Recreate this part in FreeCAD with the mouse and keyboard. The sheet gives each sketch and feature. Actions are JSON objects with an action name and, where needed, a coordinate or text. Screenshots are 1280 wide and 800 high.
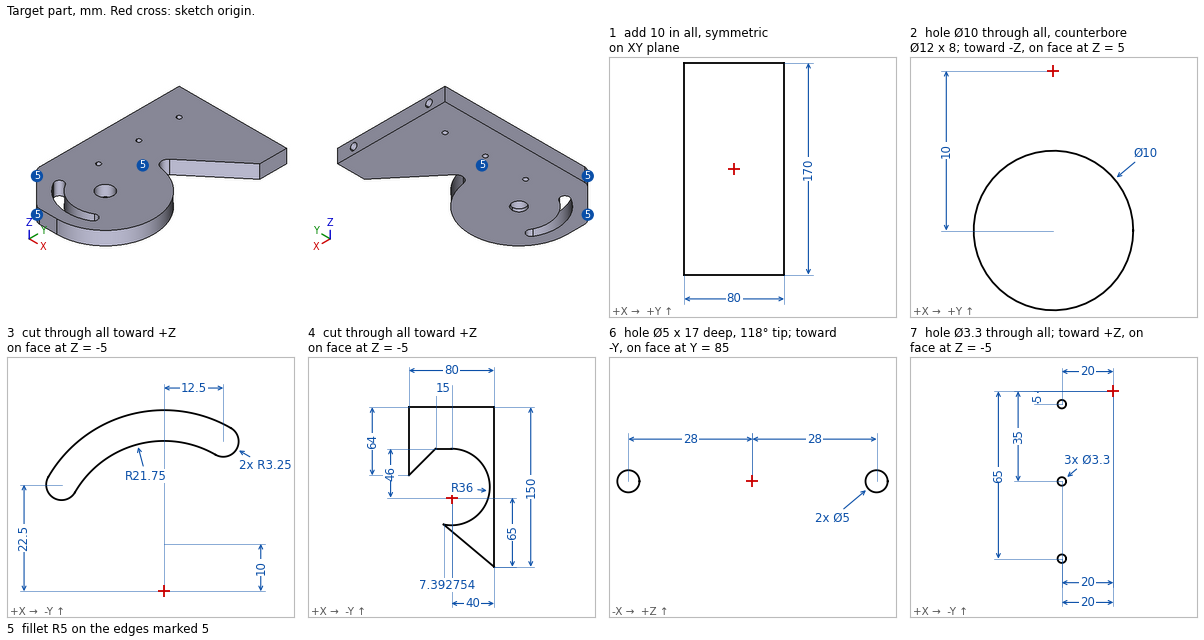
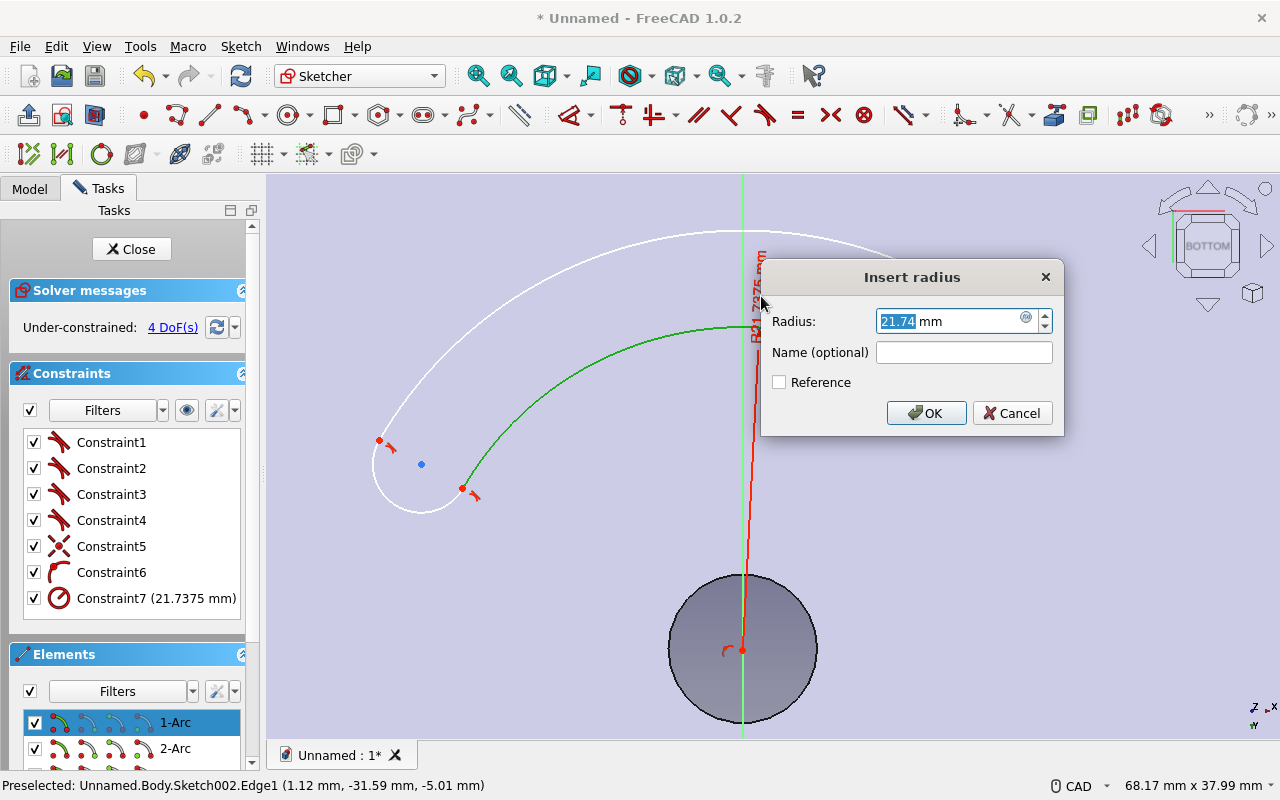
{"action": "type", "text": "21.75"}
{"action": "key", "text": "Return"}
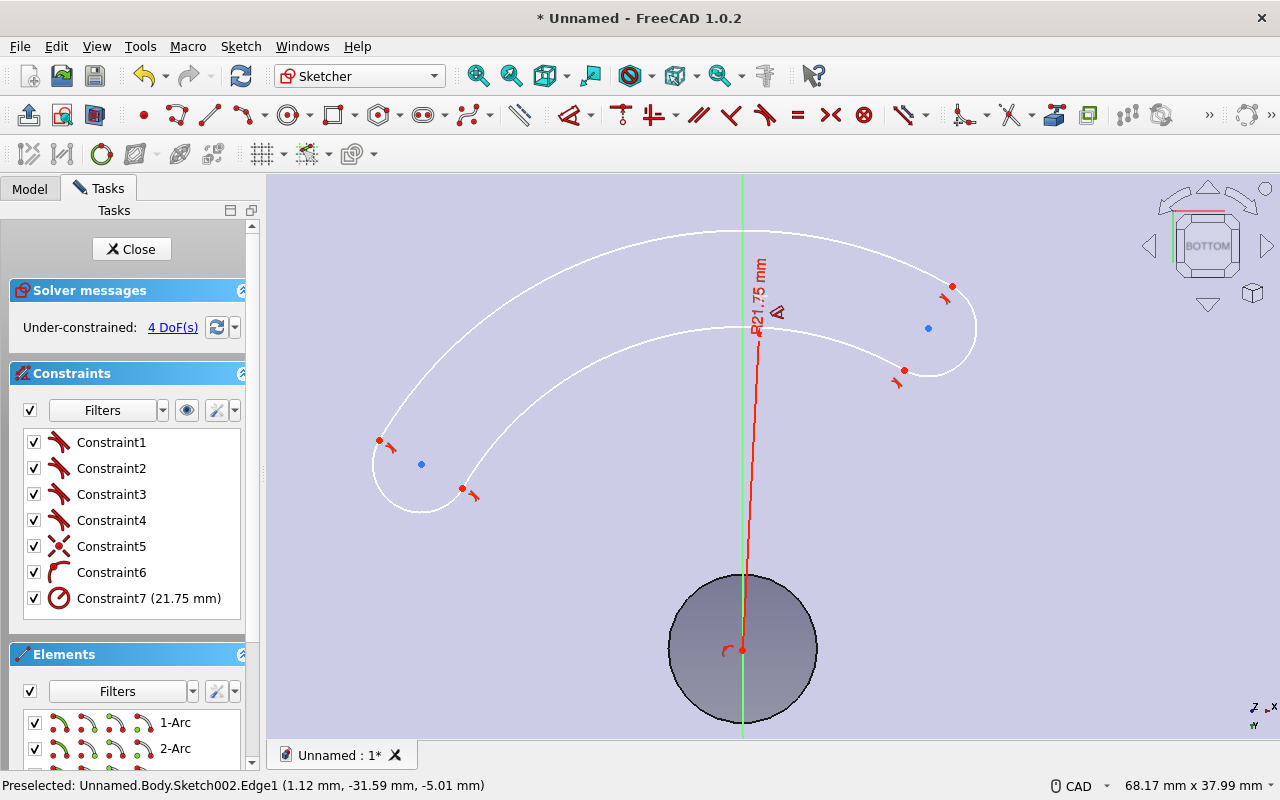
{"action": "left_click", "coordinate": [948, 372]}
{"action": "left_click", "coordinate": [961, 401]}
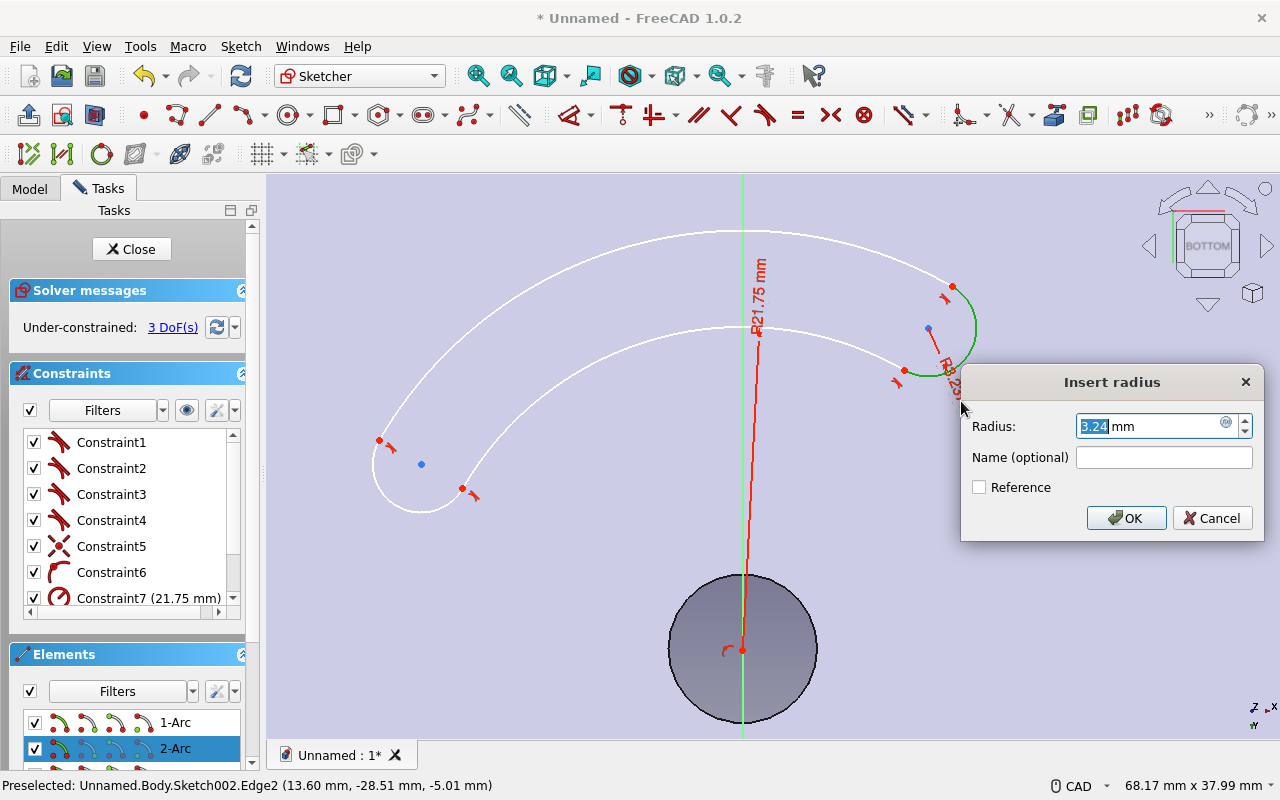
{"action": "type", "text": "3.25"}
{"action": "key", "text": "Return"}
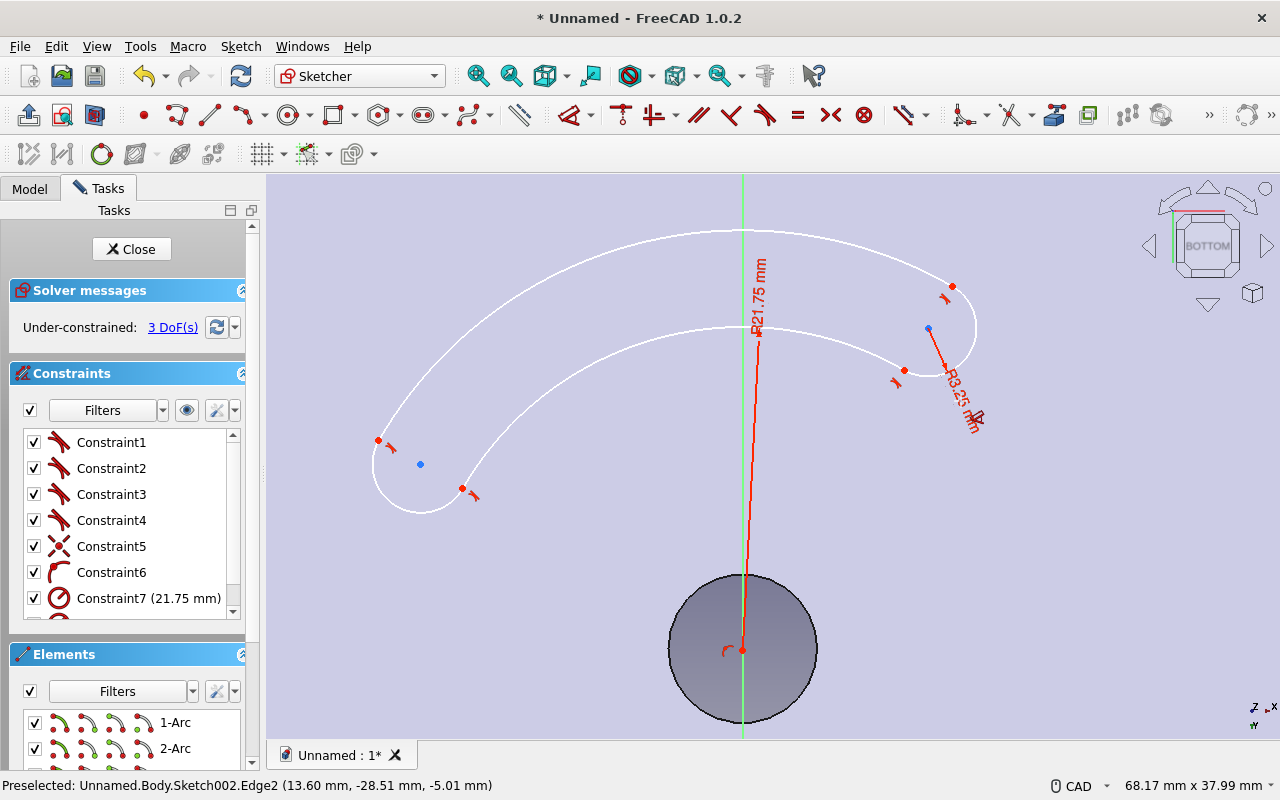
{"action": "left_click", "coordinate": [743, 650]}
{"action": "left_click", "coordinate": [777, 681]}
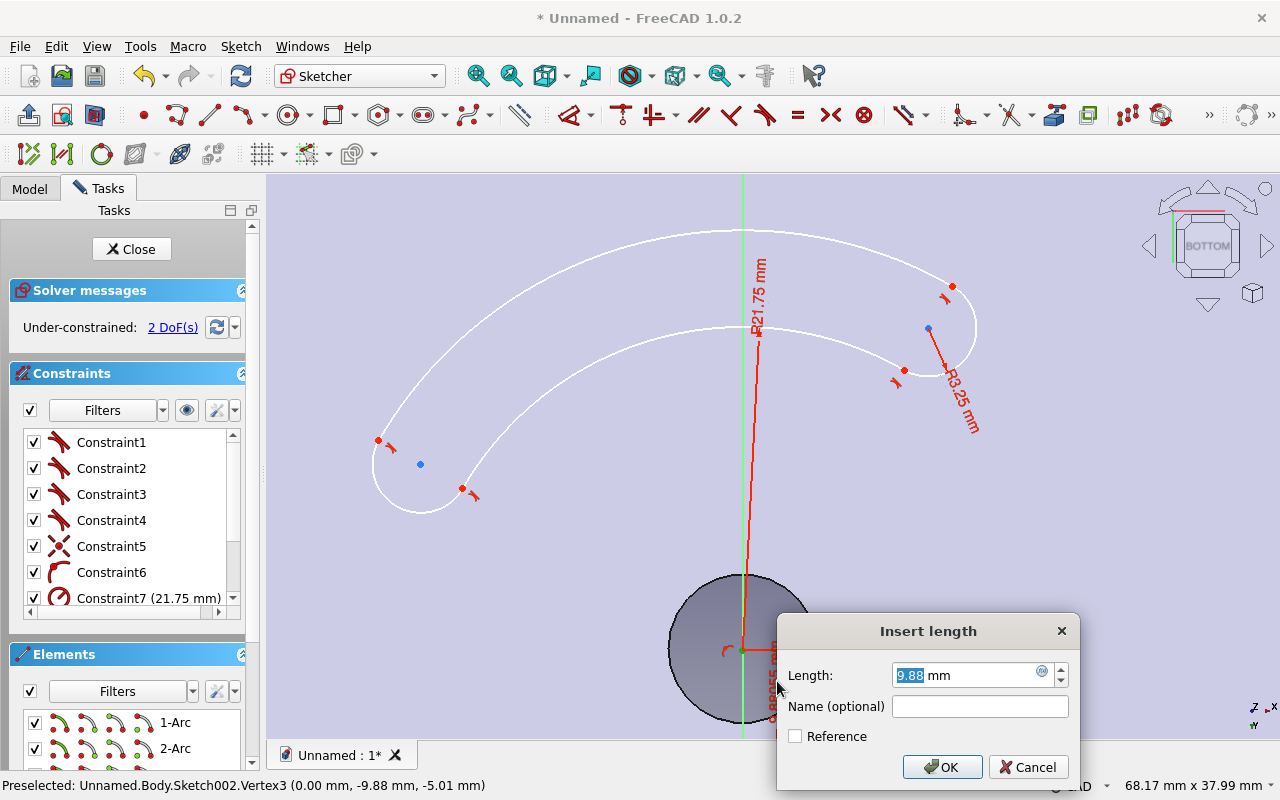
{"action": "type", "text": "10"}
{"action": "key", "text": "Return"}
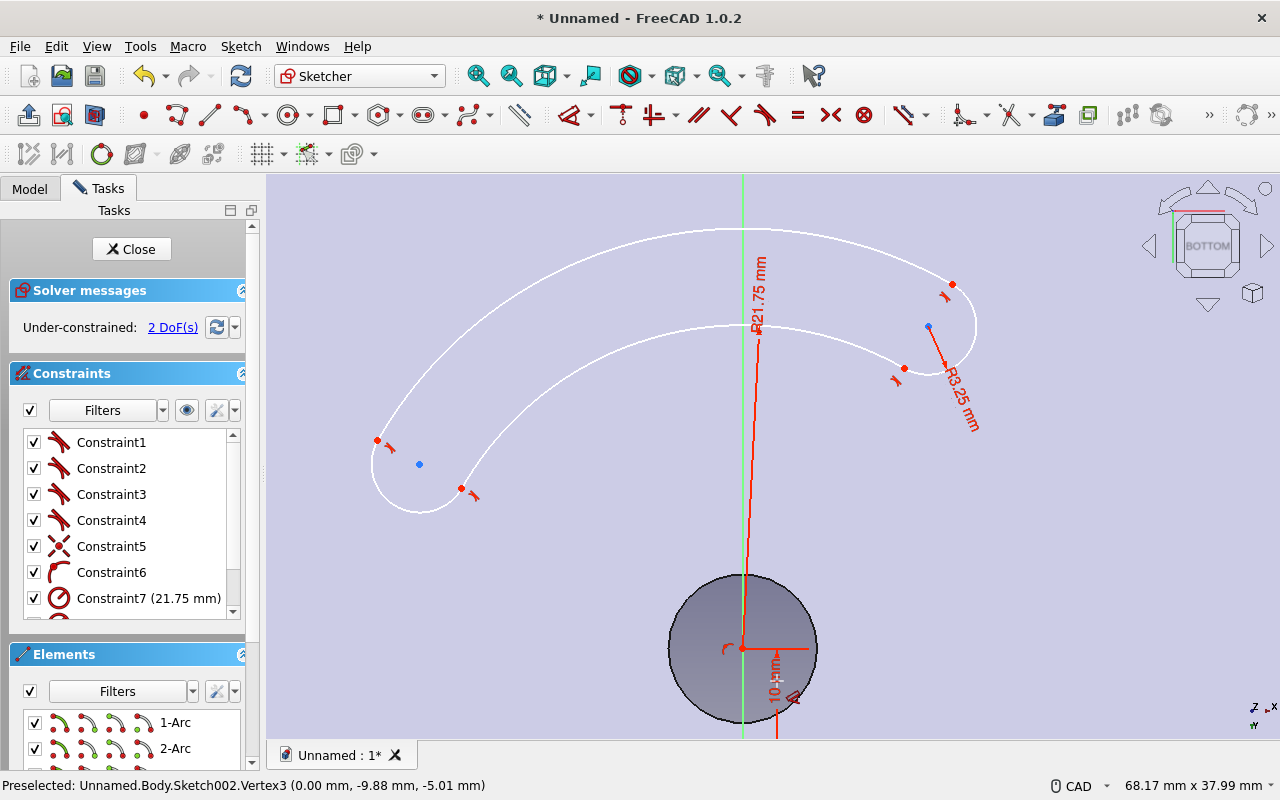
{"action": "left_click", "coordinate": [928, 326]}
{"action": "left_click", "coordinate": [835, 292]}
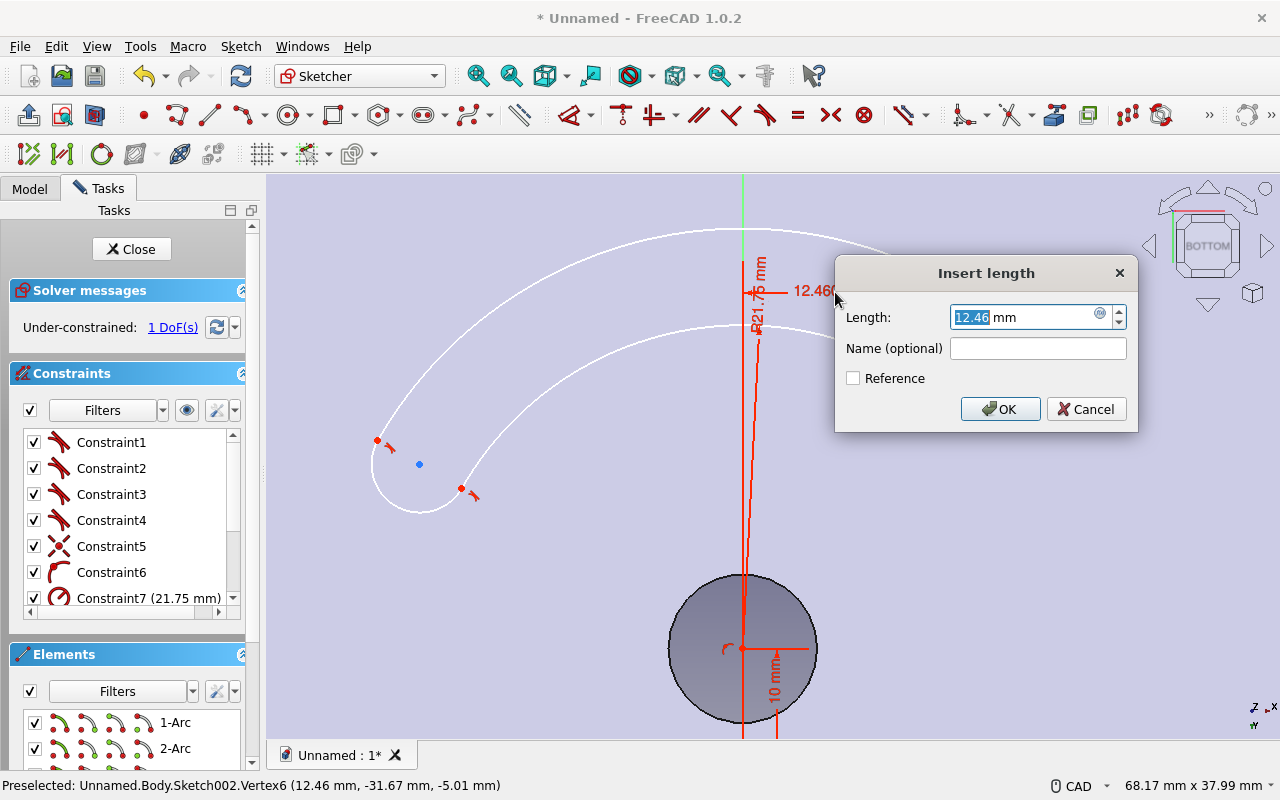
{"action": "type", "text": "12.5"}
{"action": "key", "text": "Return"}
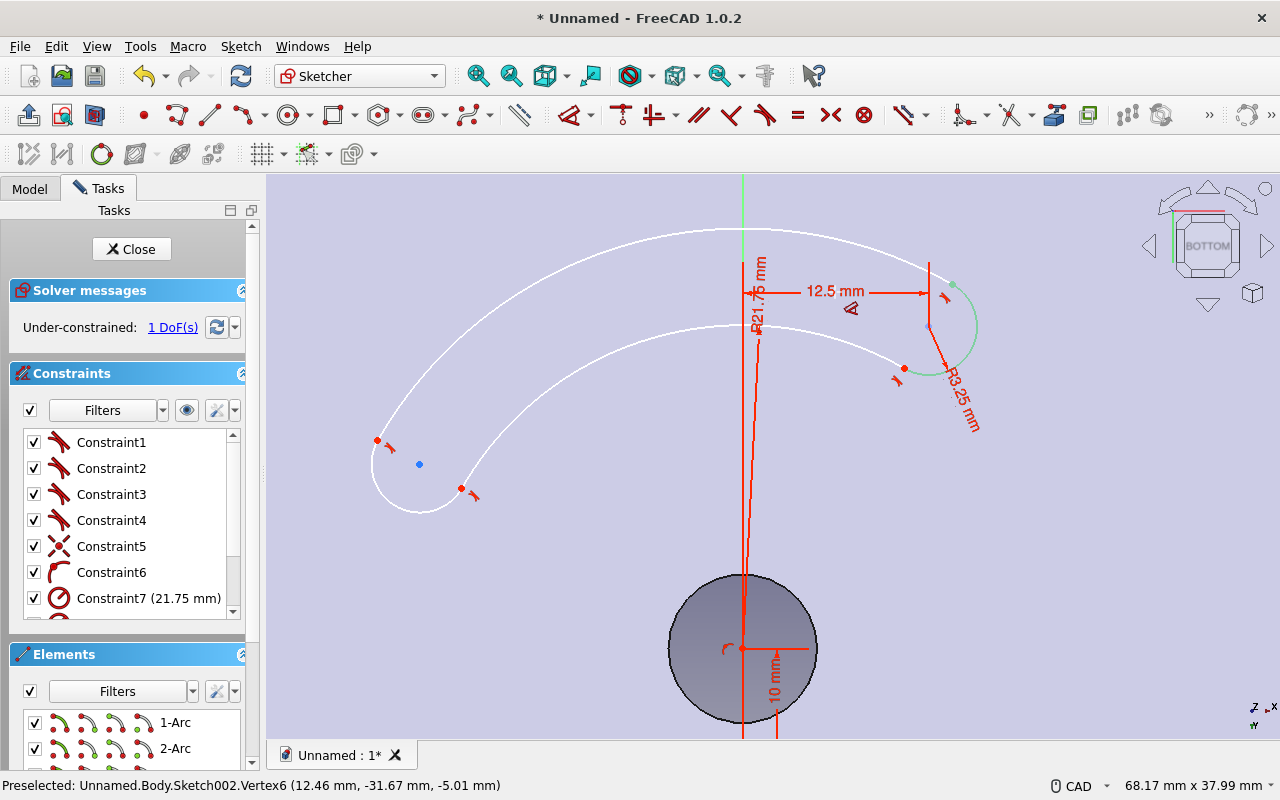
{"action": "left_click", "coordinate": [420, 464]}
{"action": "left_click", "coordinate": [386, 588]}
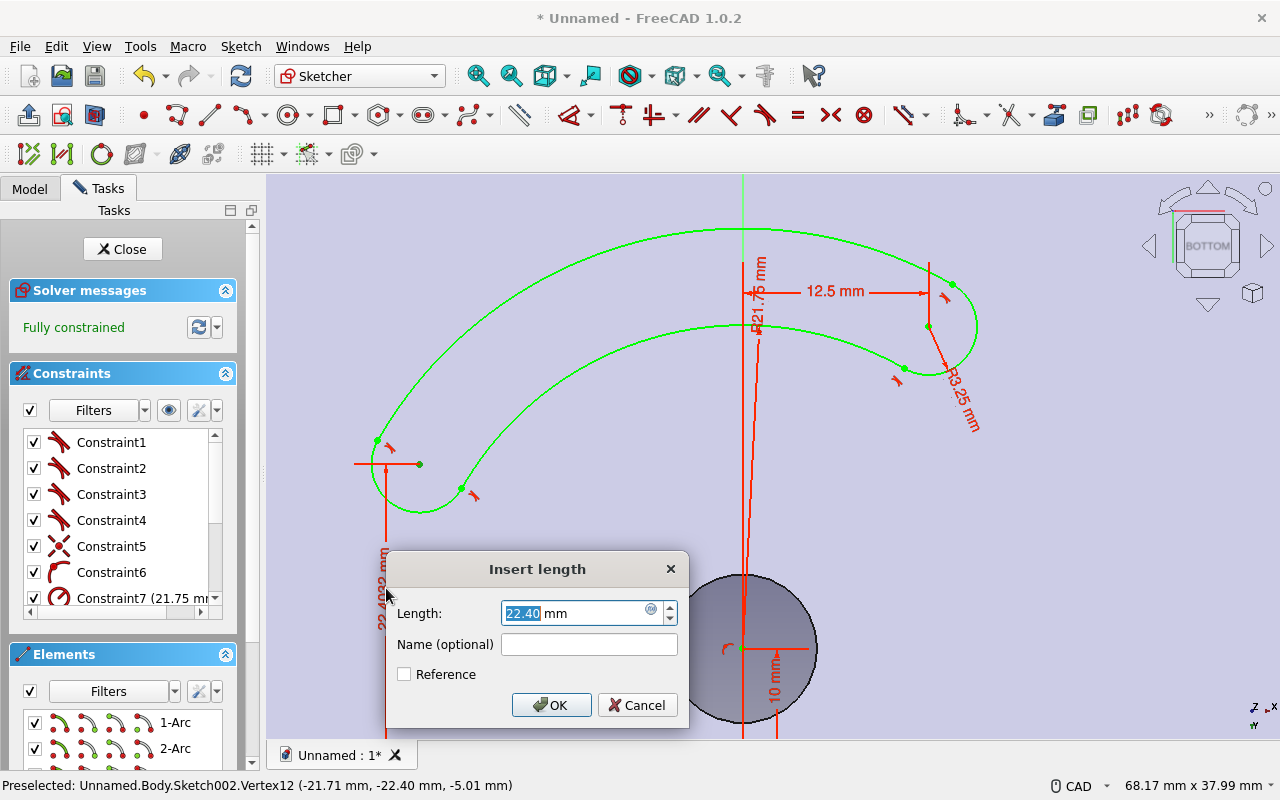
{"action": "type", "text": "22.5"}
{"action": "key", "text": "Return"}
{"action": "key", "text": "Escape"}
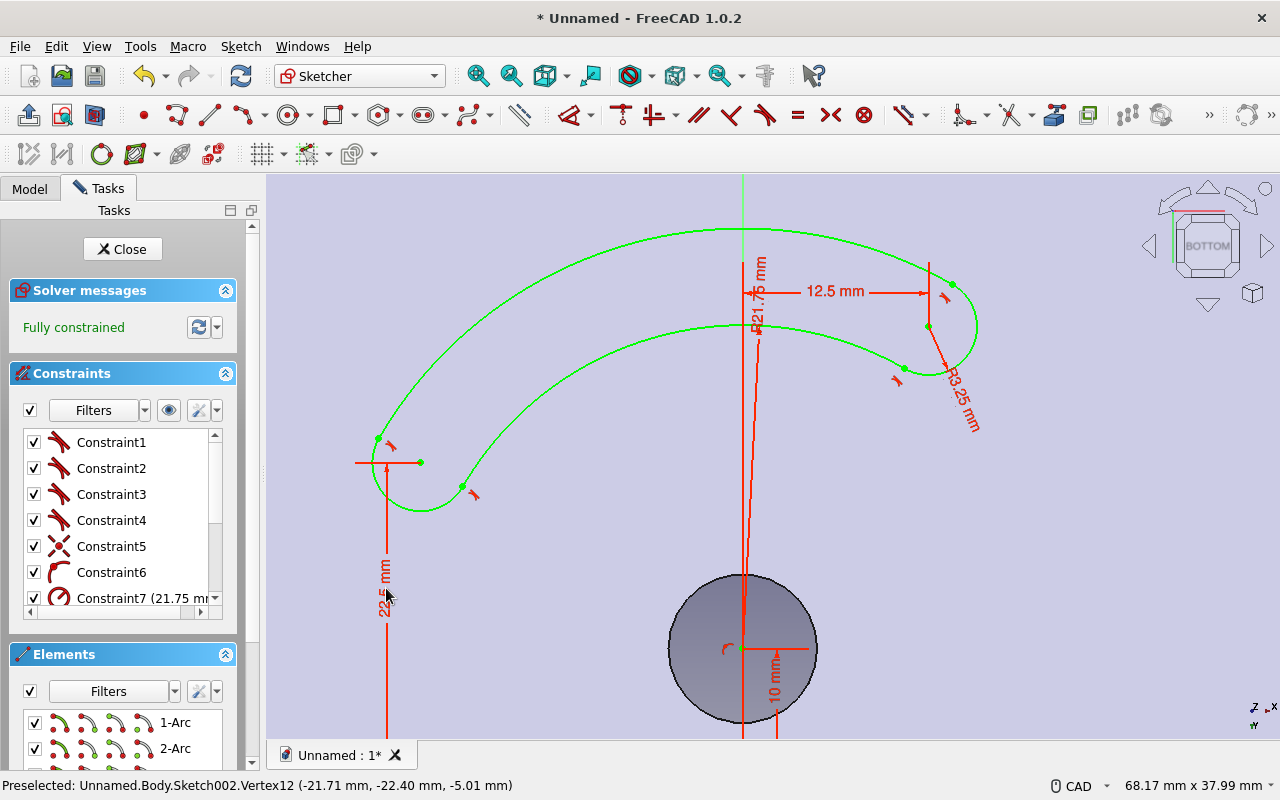
{"action": "left_click", "coordinate": [123, 249]}